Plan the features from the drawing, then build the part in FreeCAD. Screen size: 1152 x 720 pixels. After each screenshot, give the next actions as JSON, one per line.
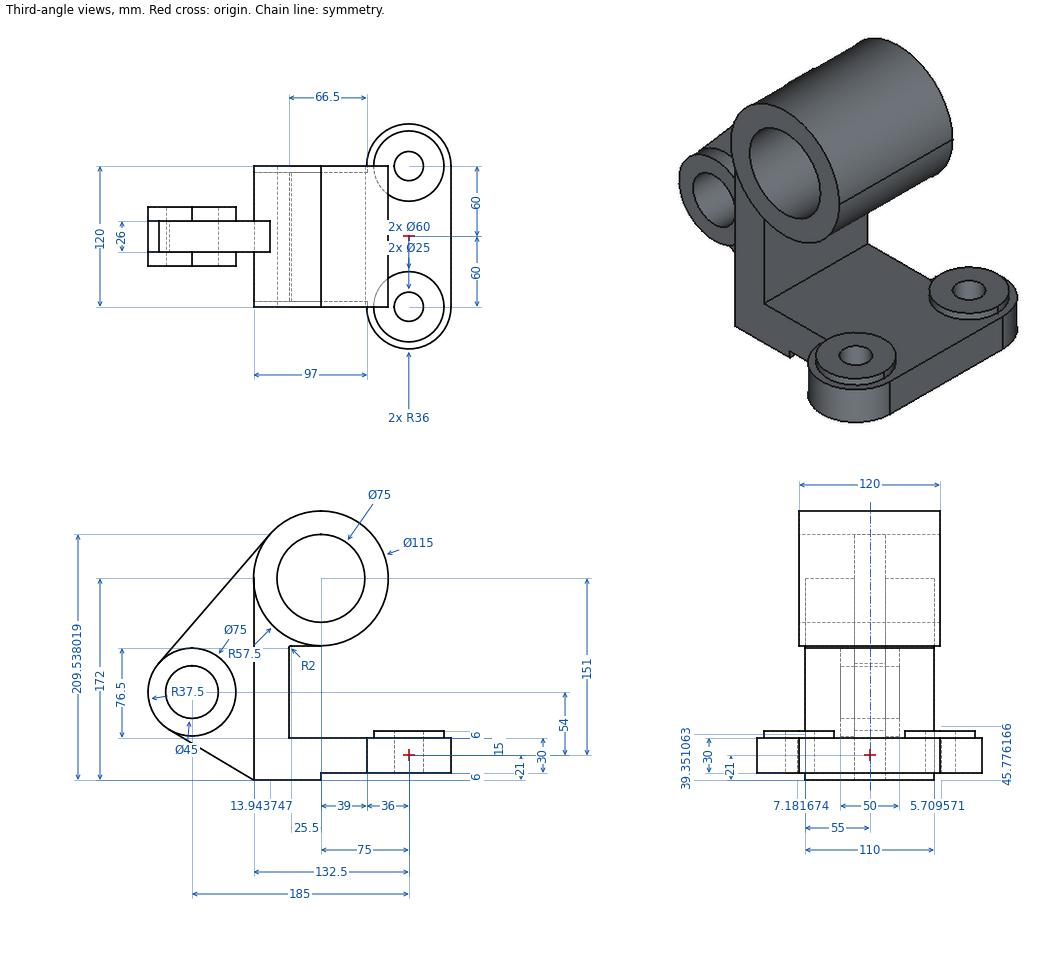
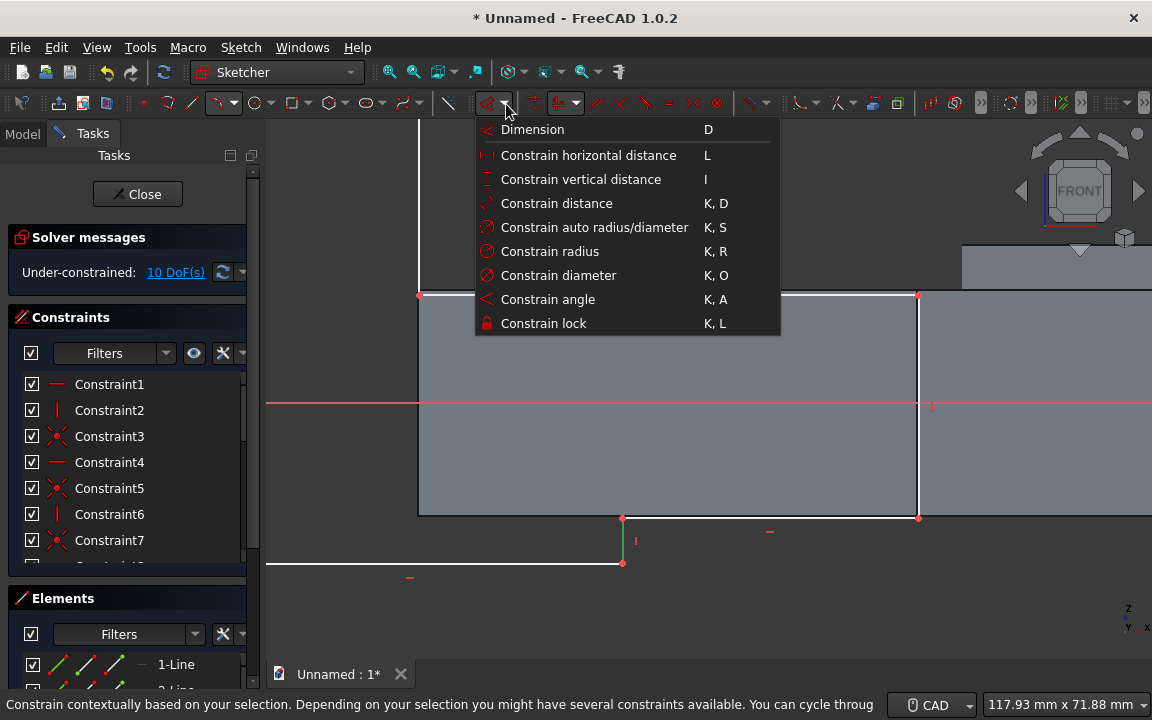
{"action": "left_click", "coordinate": [628, 179]}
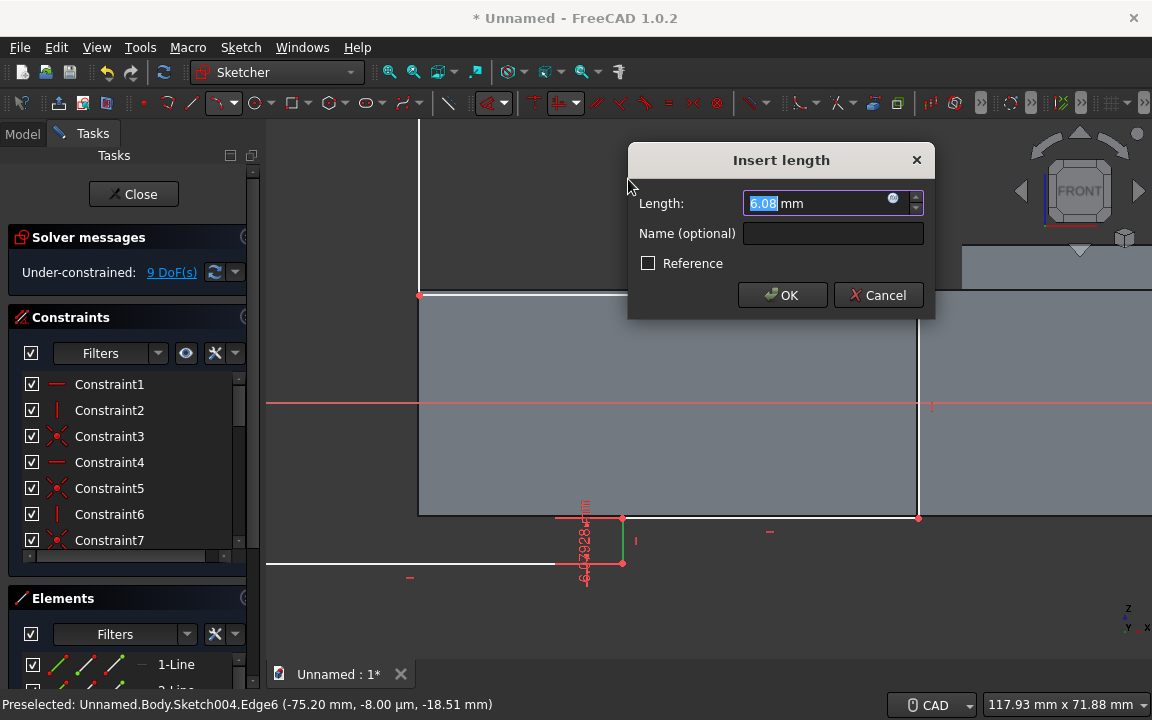
{"action": "type", "text": "6"}
{"action": "key", "text": "Return"}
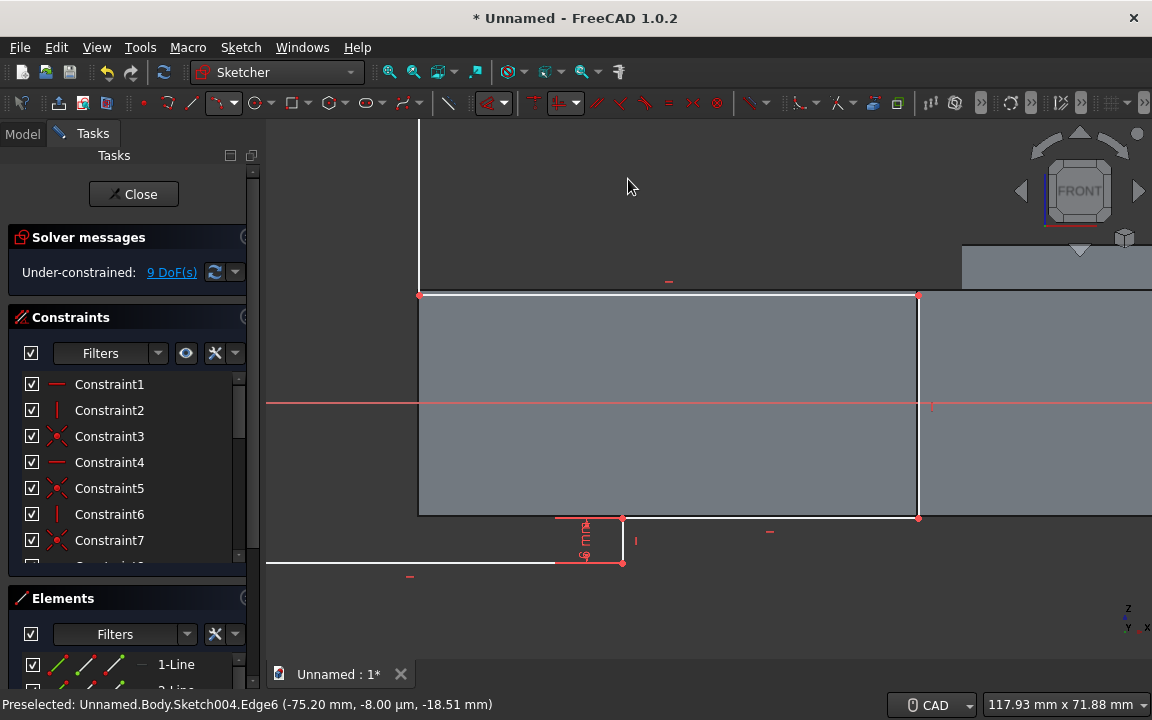
{"action": "scroll", "coordinate": [624, 544], "scroll_direction": "down", "scroll_amount": 7}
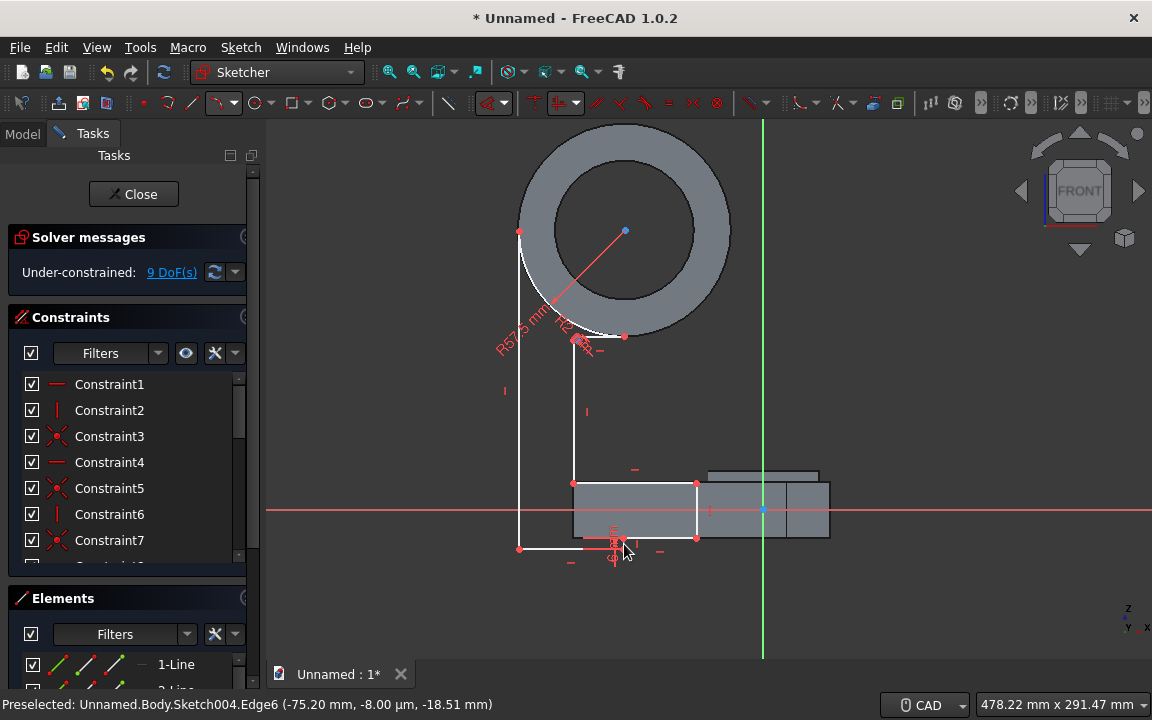
{"action": "scroll", "coordinate": [697, 500], "scroll_direction": "up", "scroll_amount": 2}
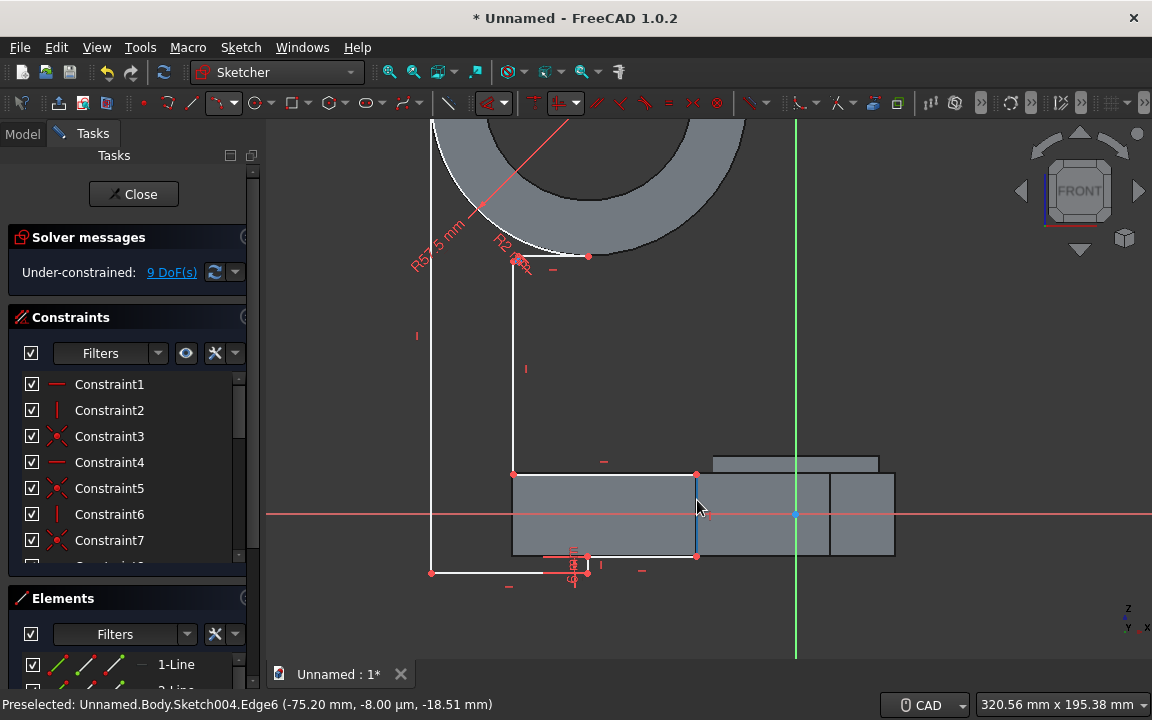
{"action": "left_click", "coordinate": [697, 499]}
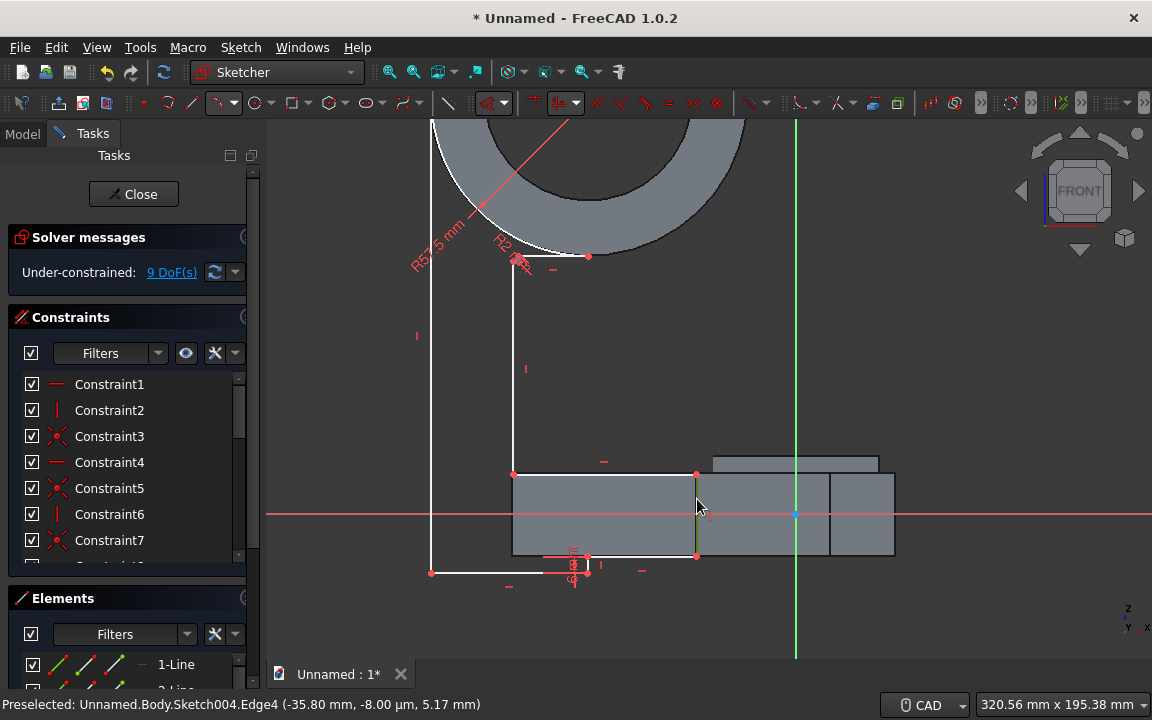
{"action": "key", "text": "i"}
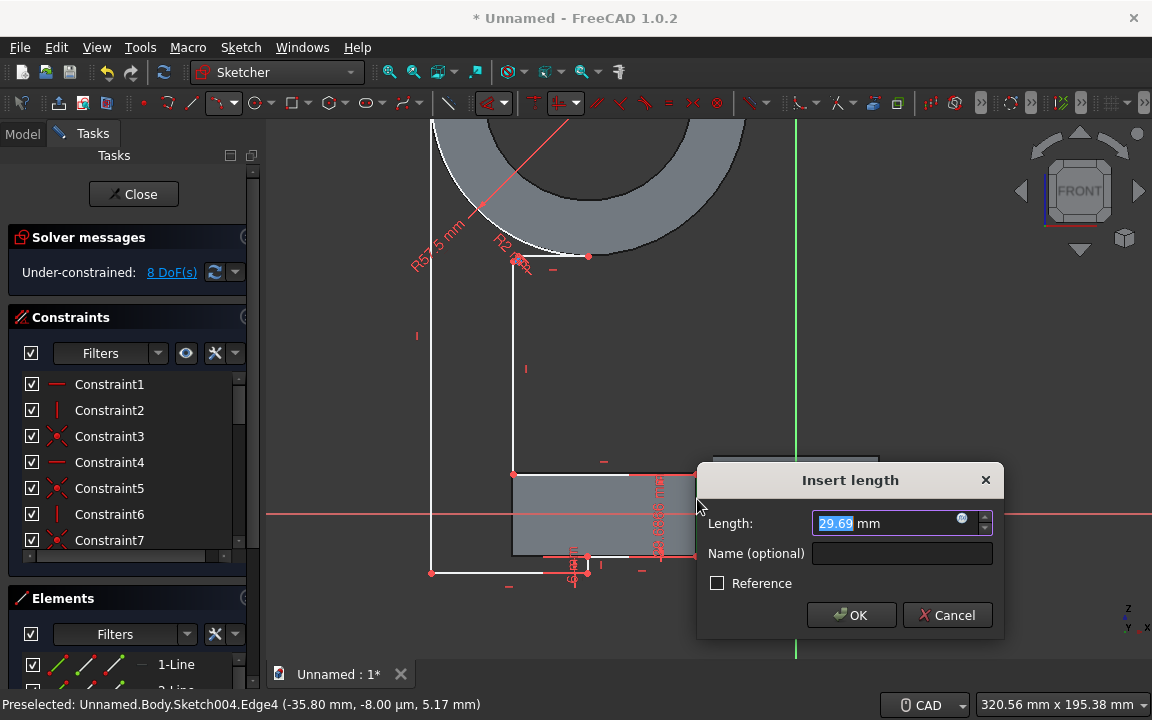
{"action": "type", "text": "30"}
{"action": "key", "text": "Return"}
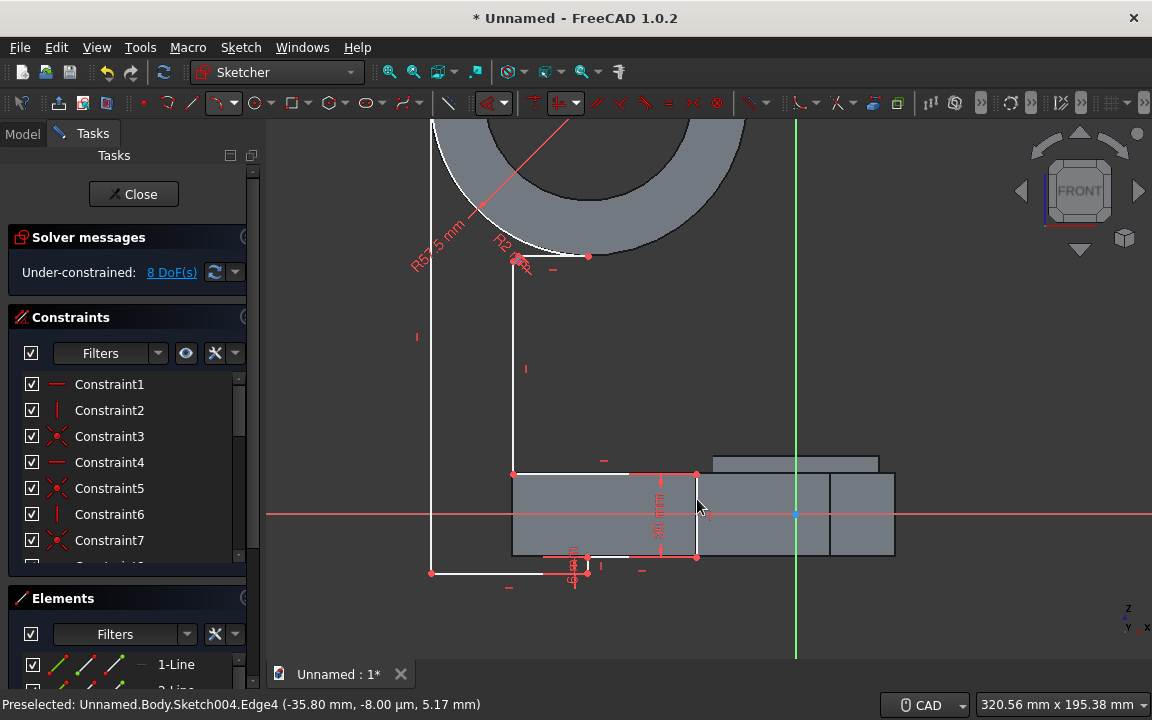
{"action": "left_click", "coordinate": [664, 557]}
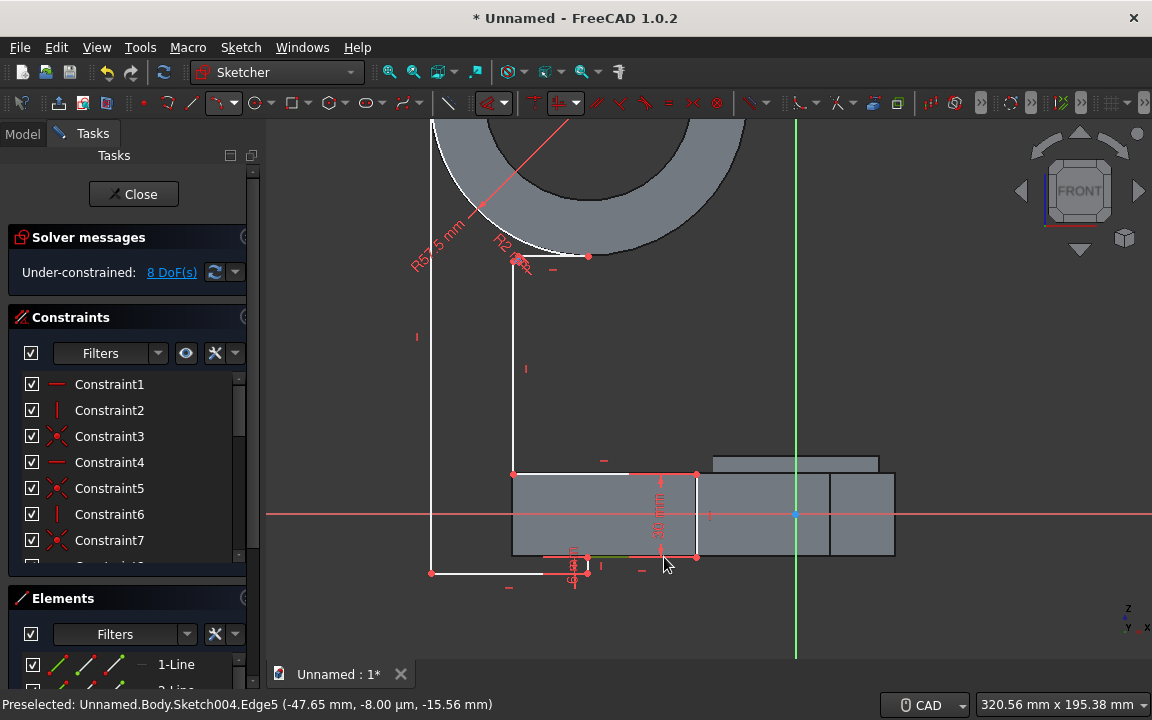
{"action": "key", "text": "l"}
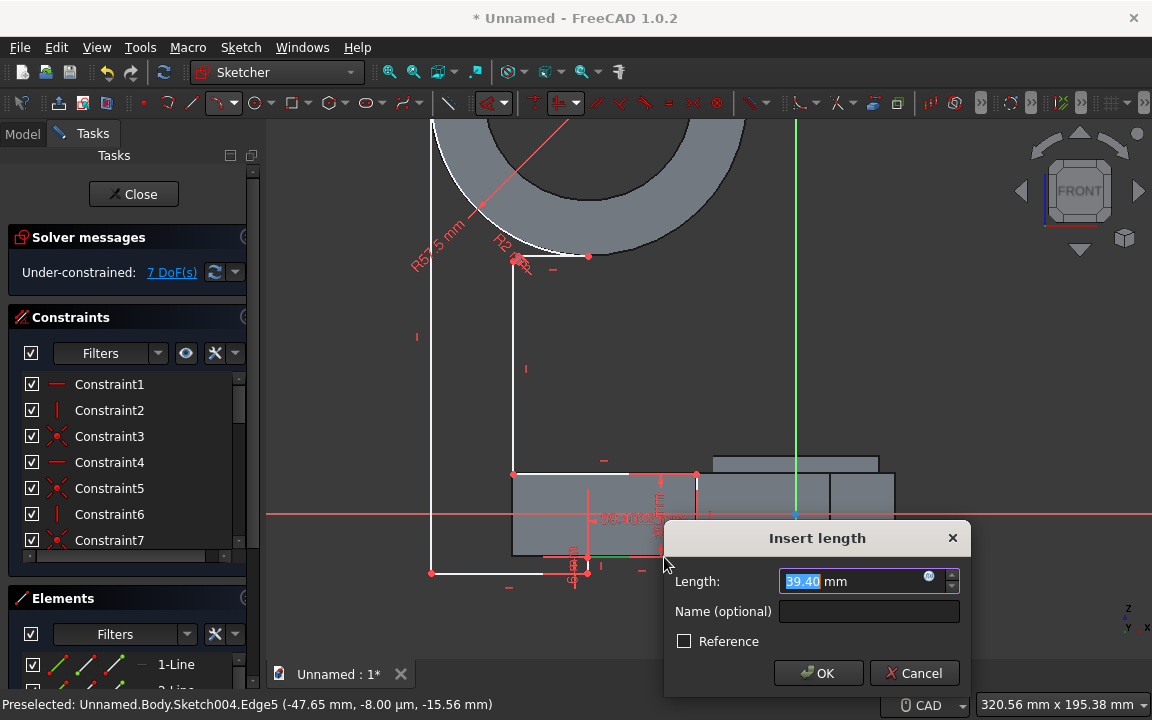
{"action": "type", "text": "39"}
{"action": "key", "text": "Return"}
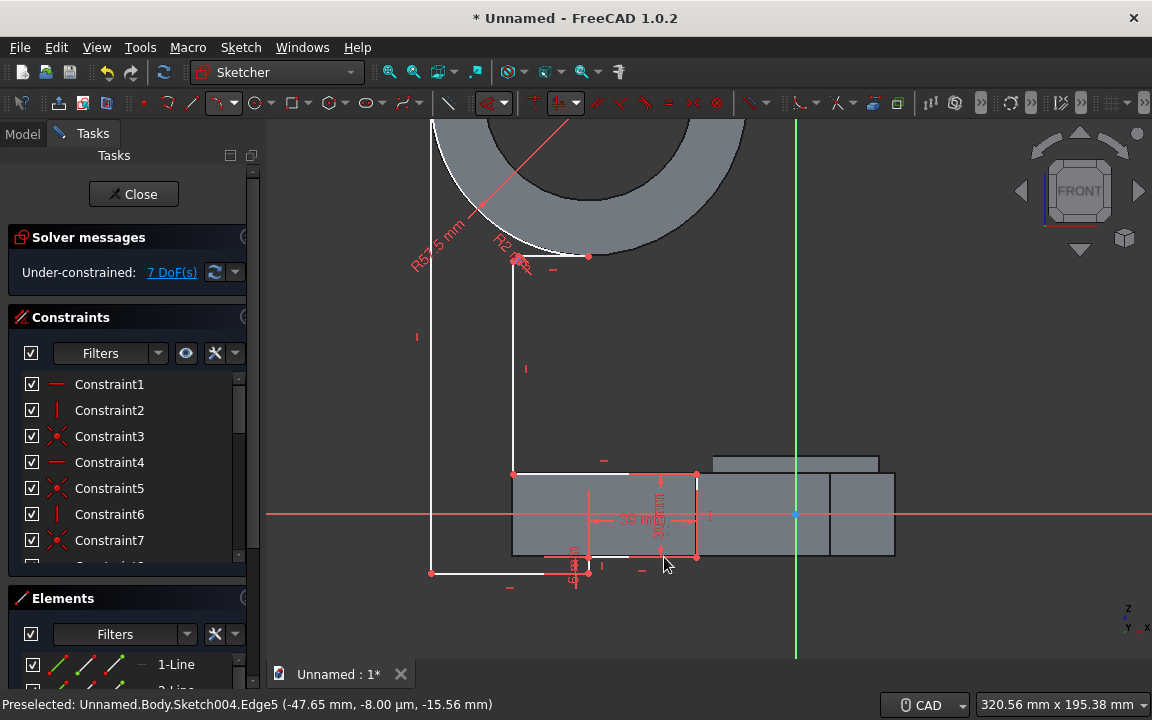
{"action": "left_click", "coordinate": [431, 431]}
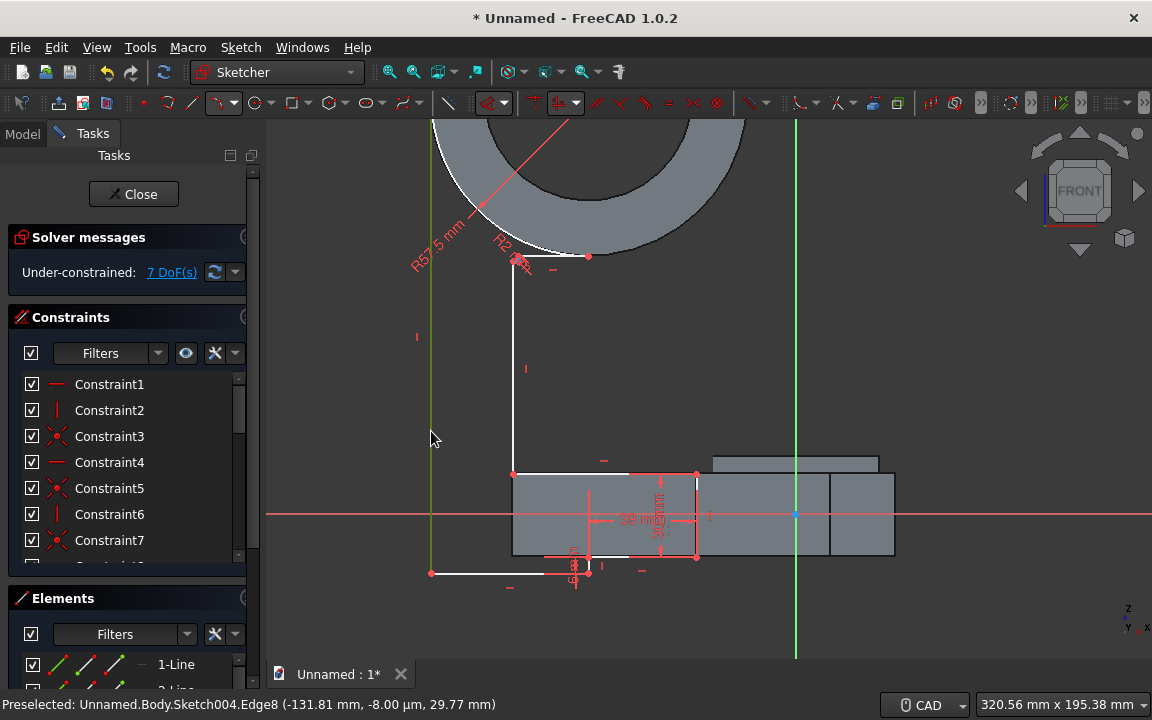
{"action": "key", "text": "i"}